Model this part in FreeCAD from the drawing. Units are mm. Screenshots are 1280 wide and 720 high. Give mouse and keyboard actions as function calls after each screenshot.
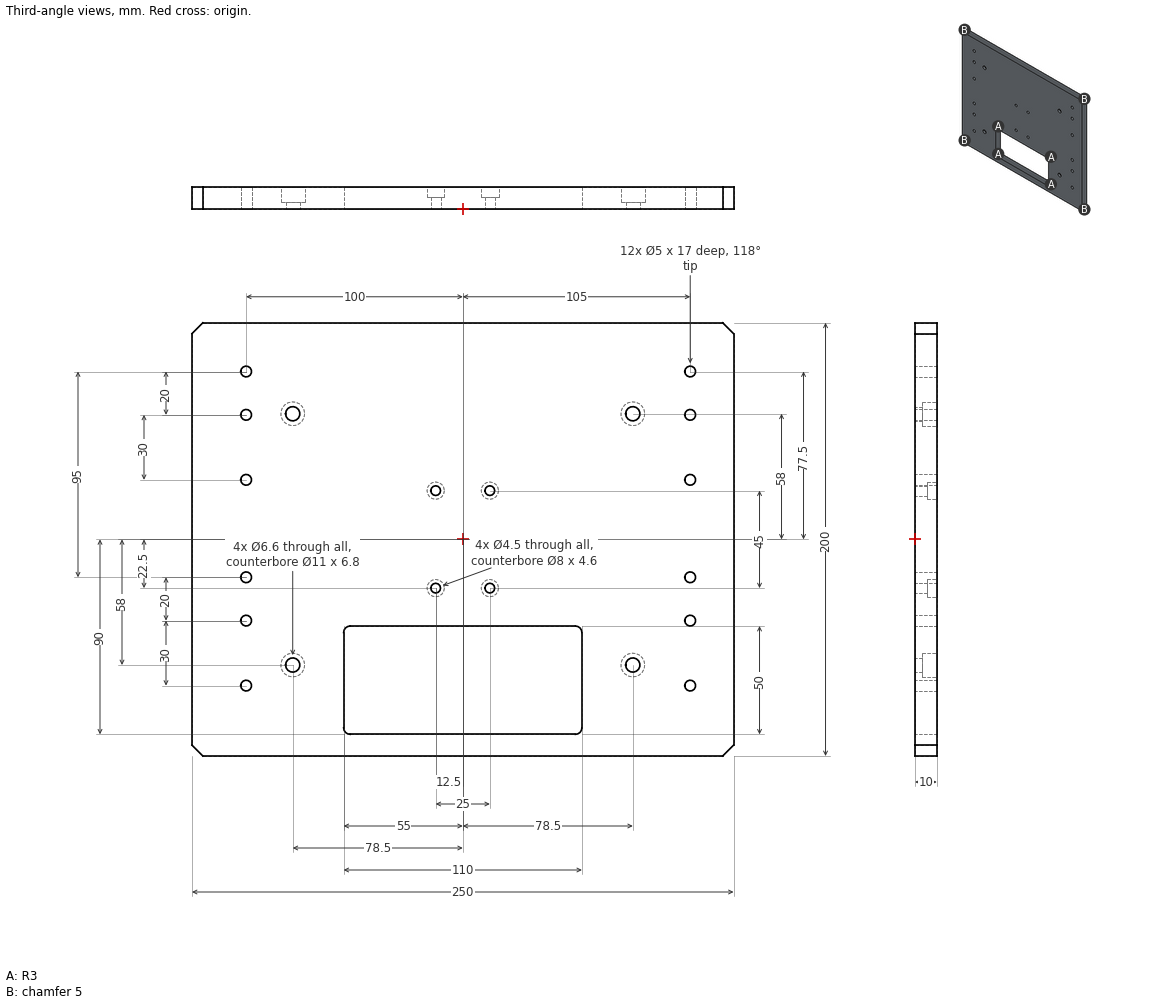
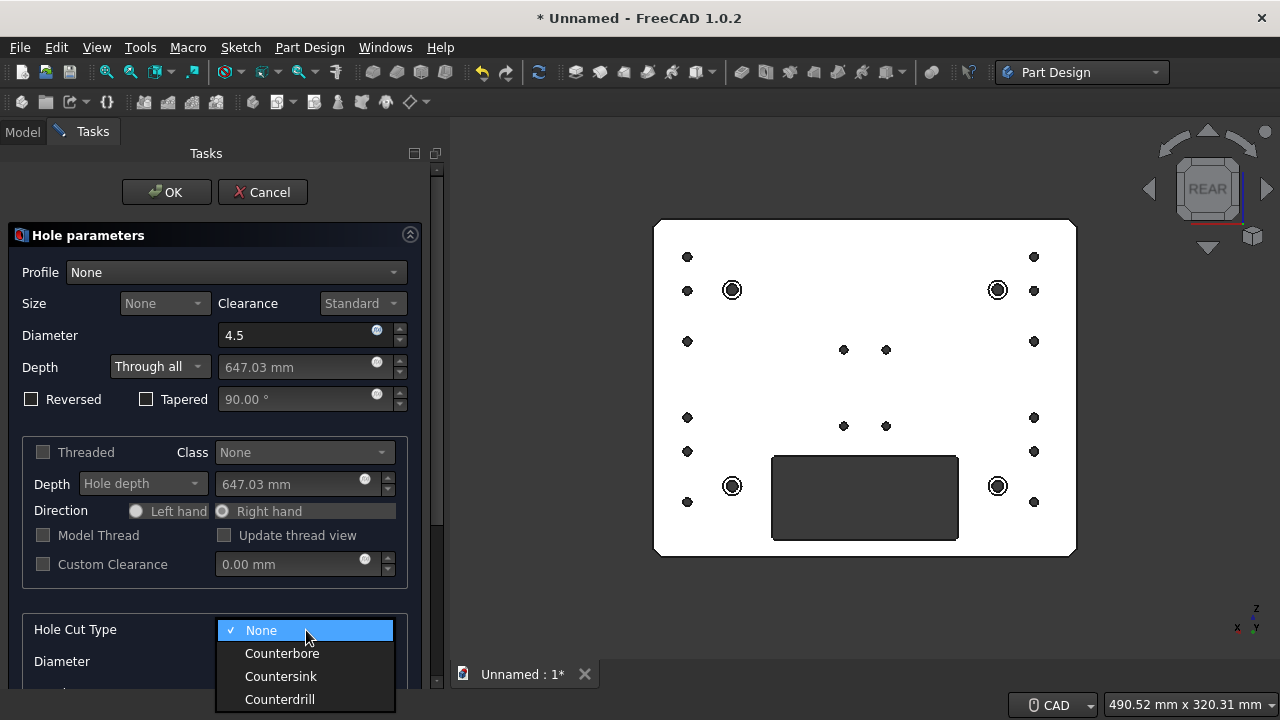
click(304, 654)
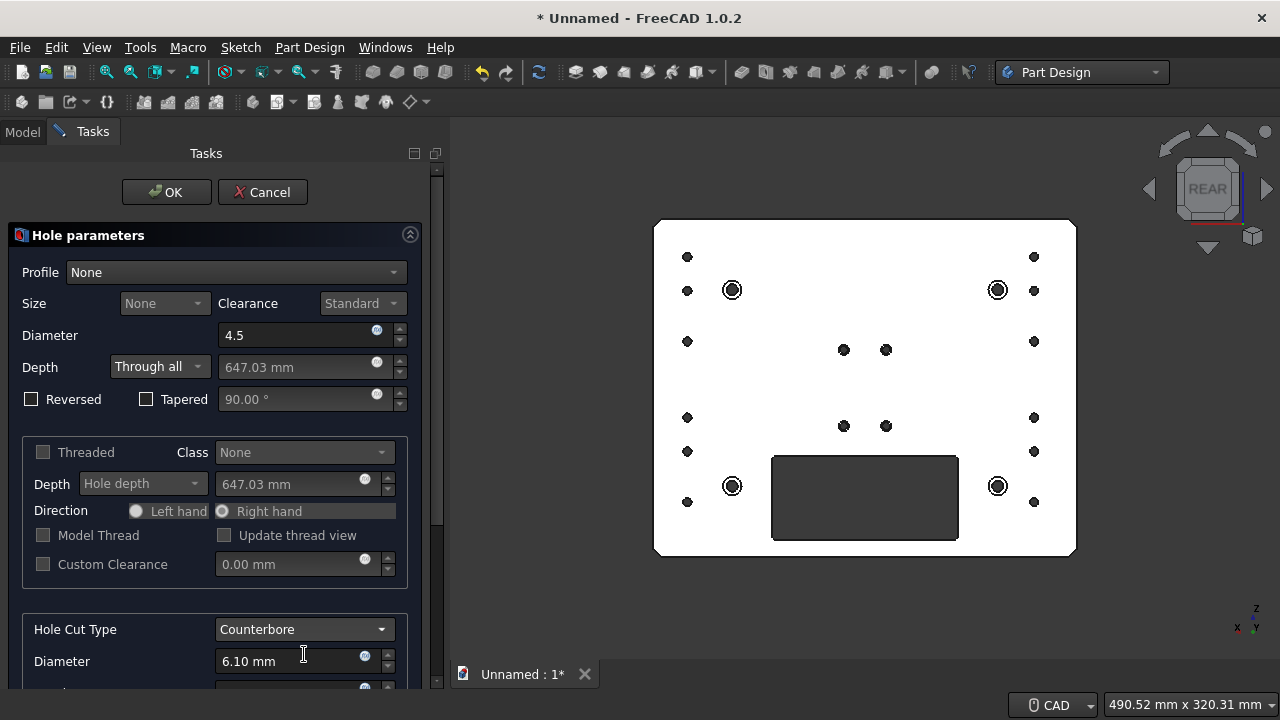
triple_click(298, 661)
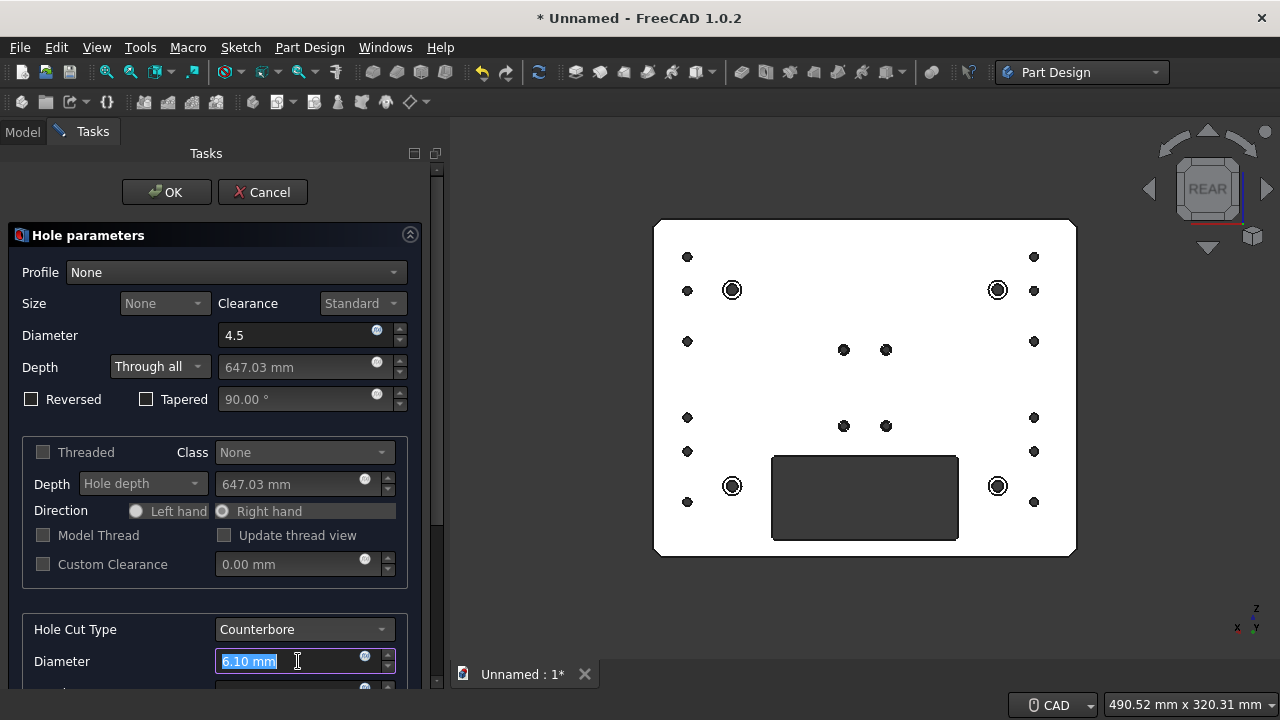
text(8)
key(Tab)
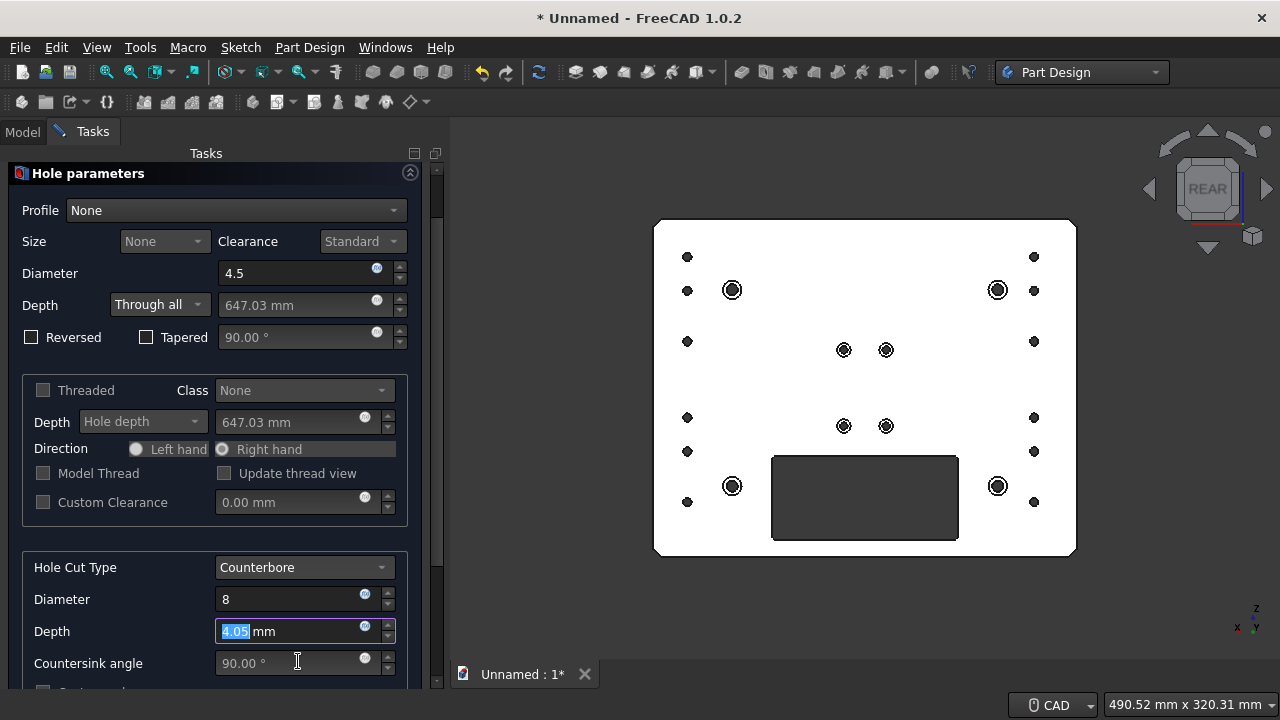
text(4.6)
key(Tab)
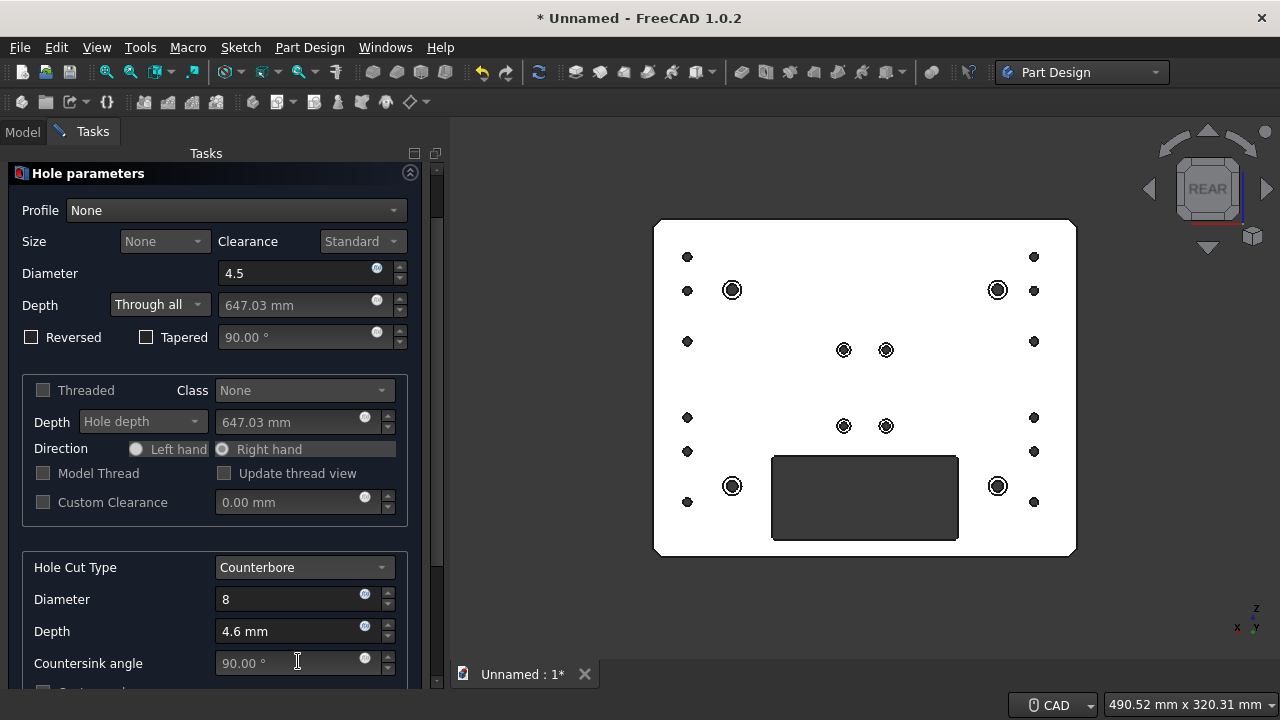
scroll(437, 426, up, 2)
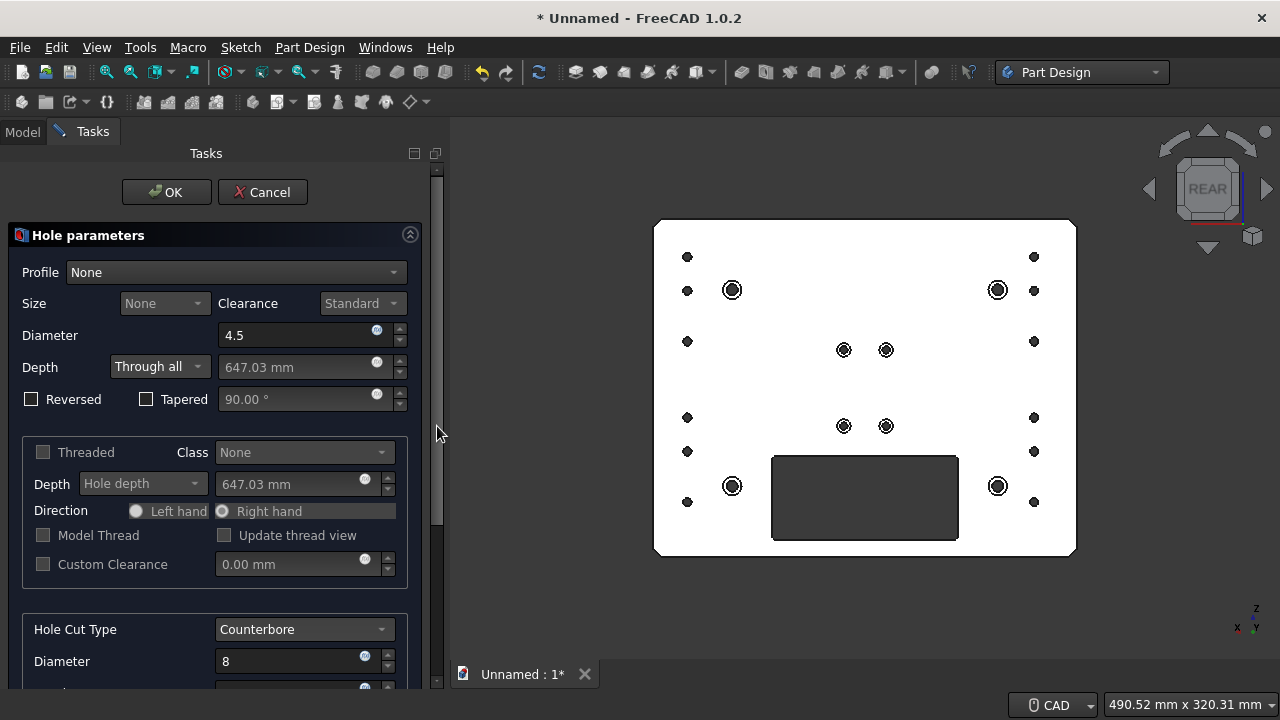
click(167, 192)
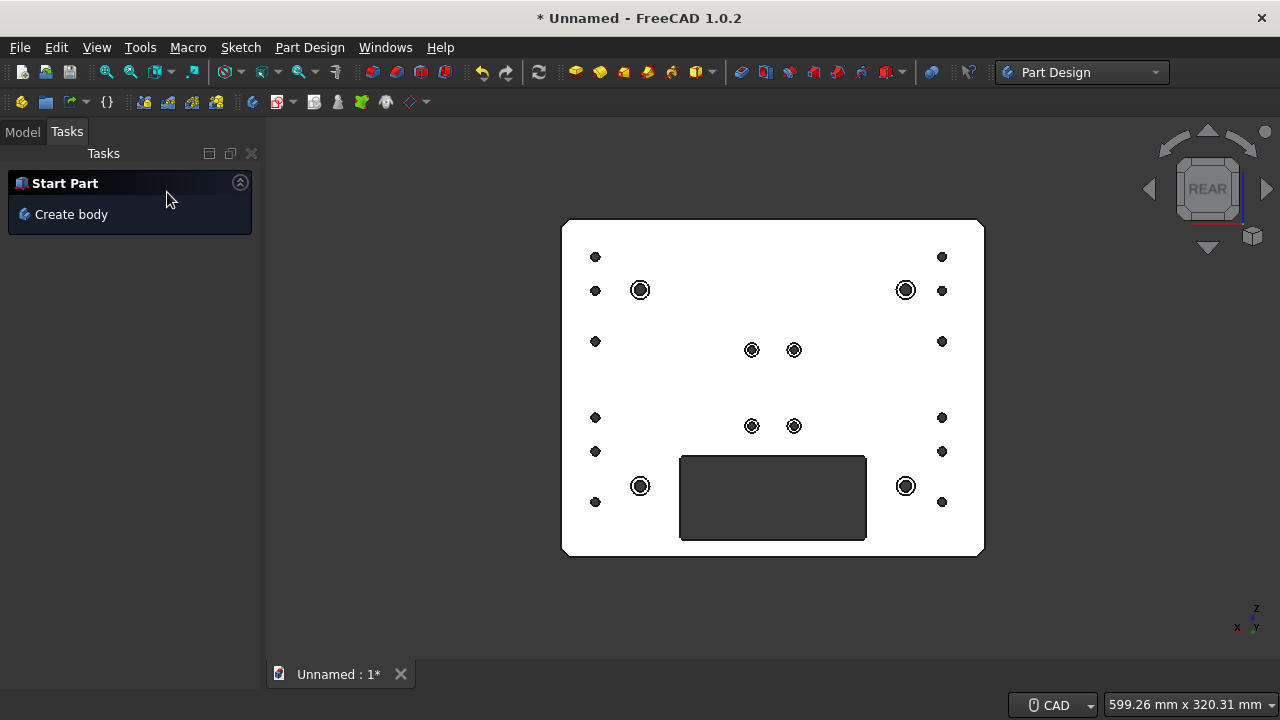
key(0)